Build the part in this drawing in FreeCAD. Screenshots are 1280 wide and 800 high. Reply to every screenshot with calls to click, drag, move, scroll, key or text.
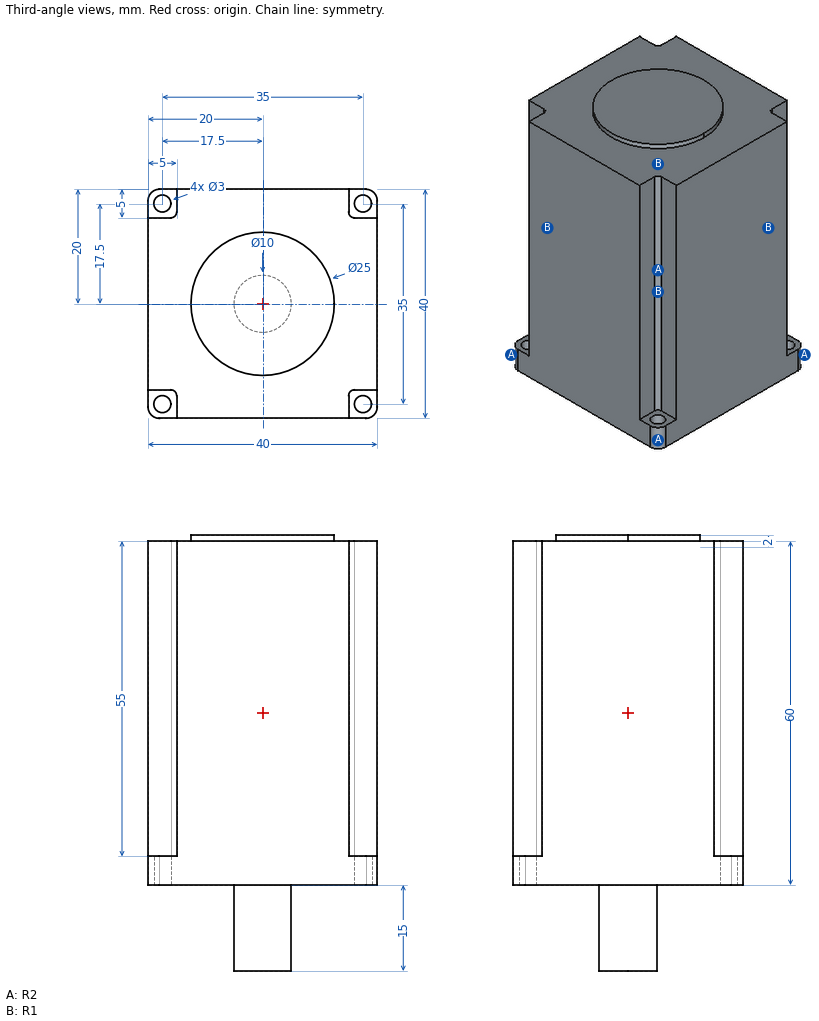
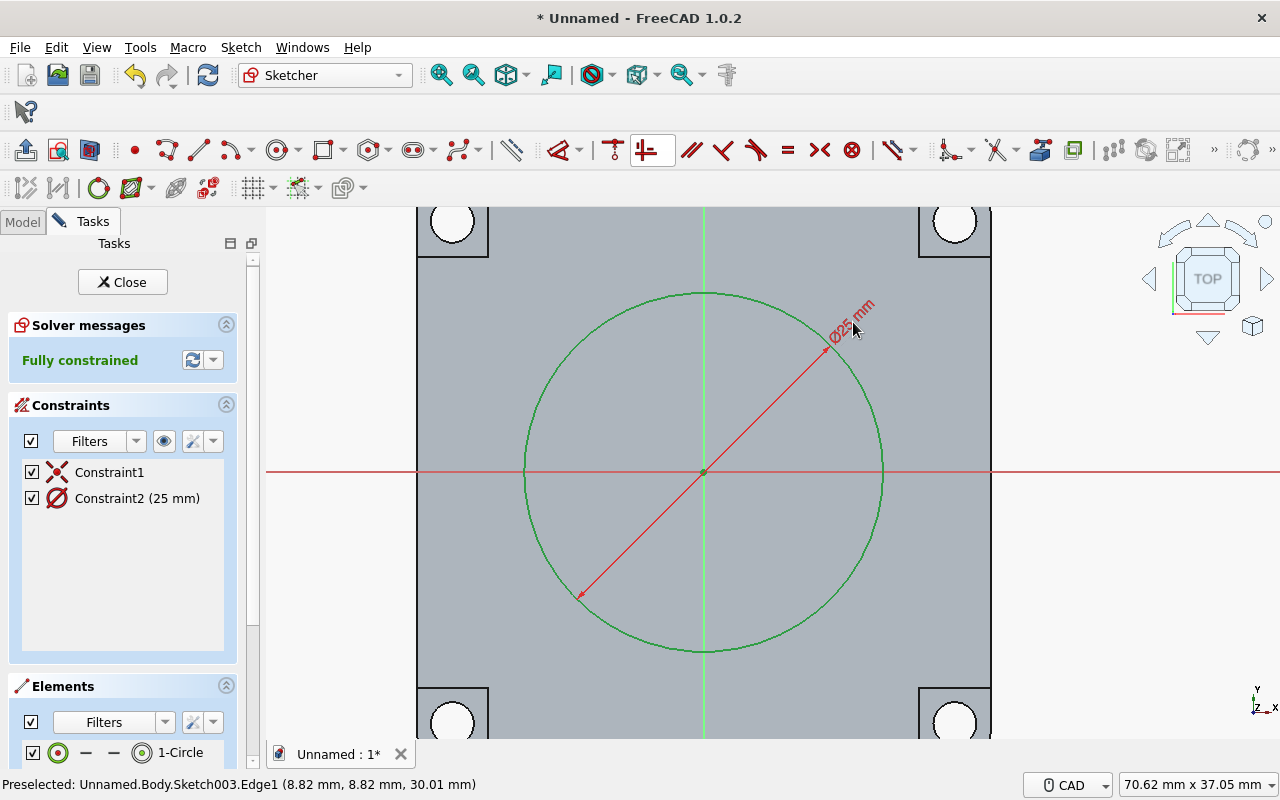
click(123, 282)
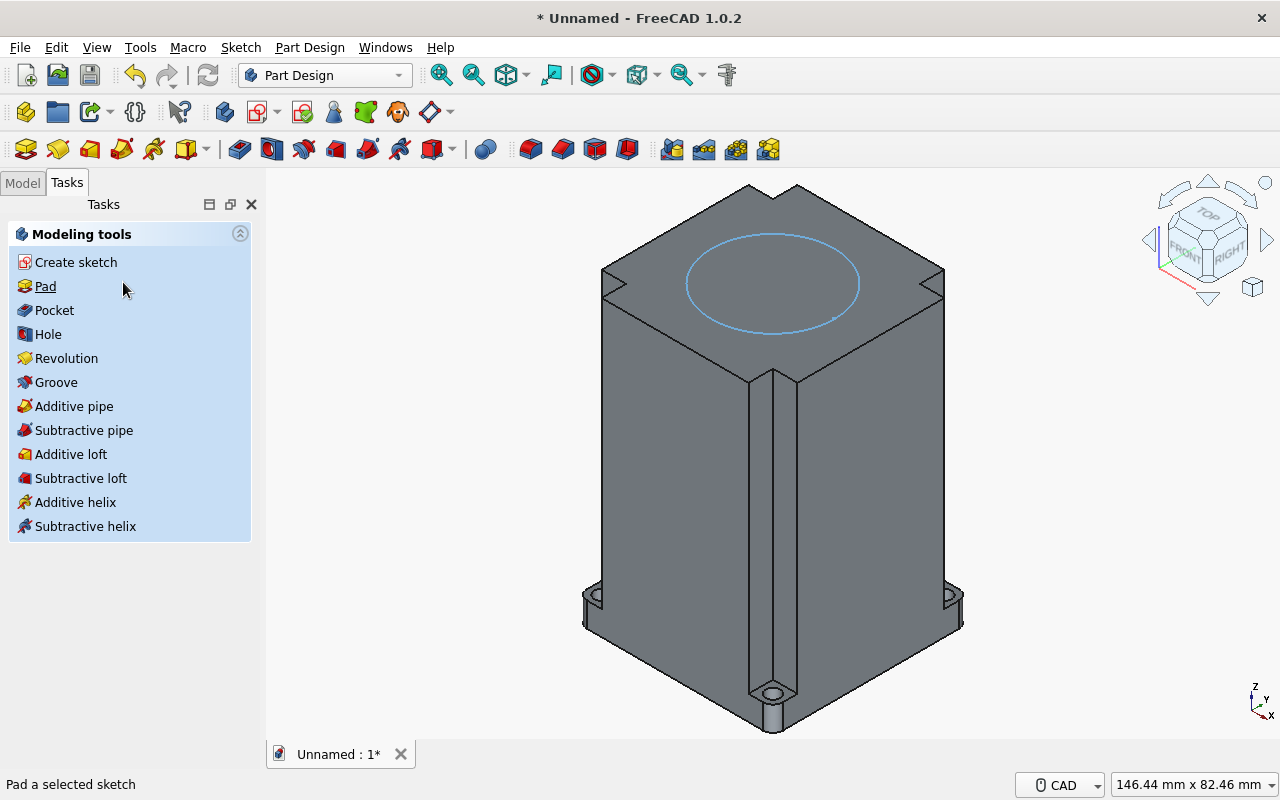
click(26, 150)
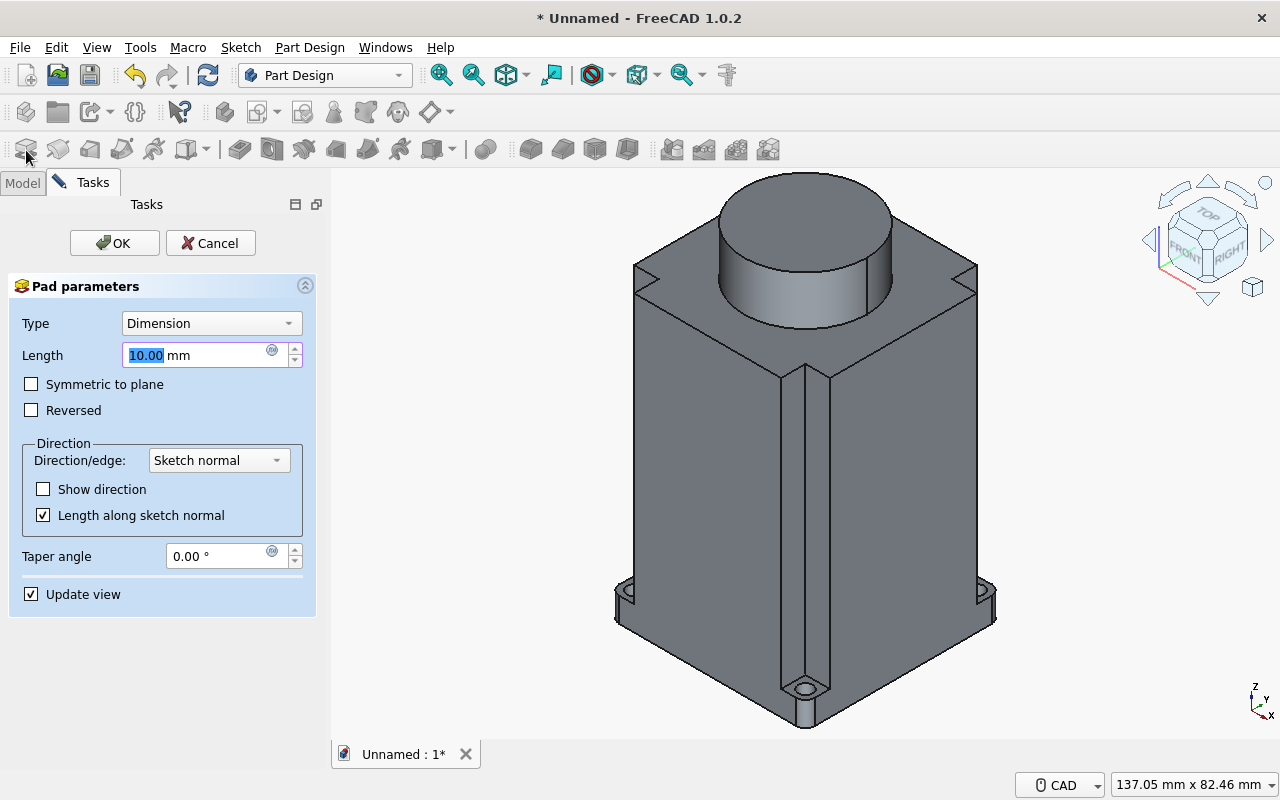
text(2)
key(Tab)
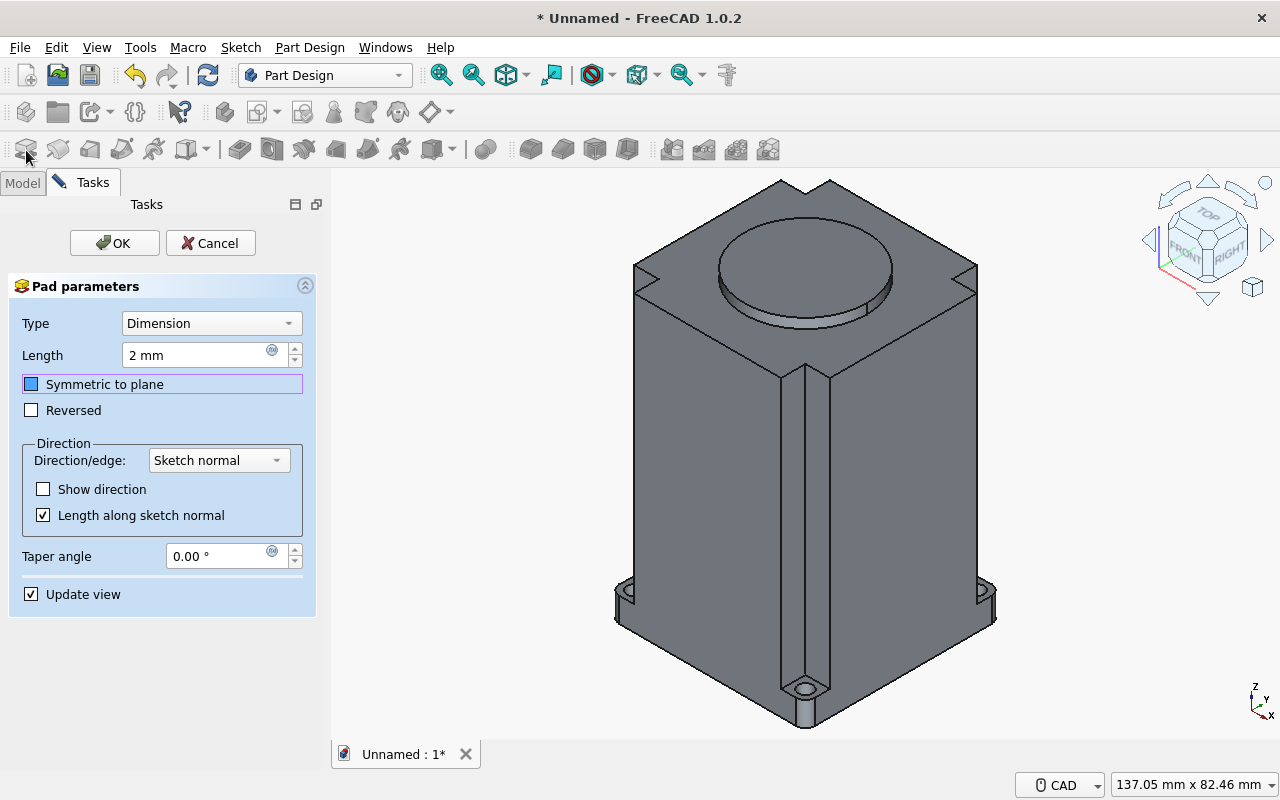
click(30, 384)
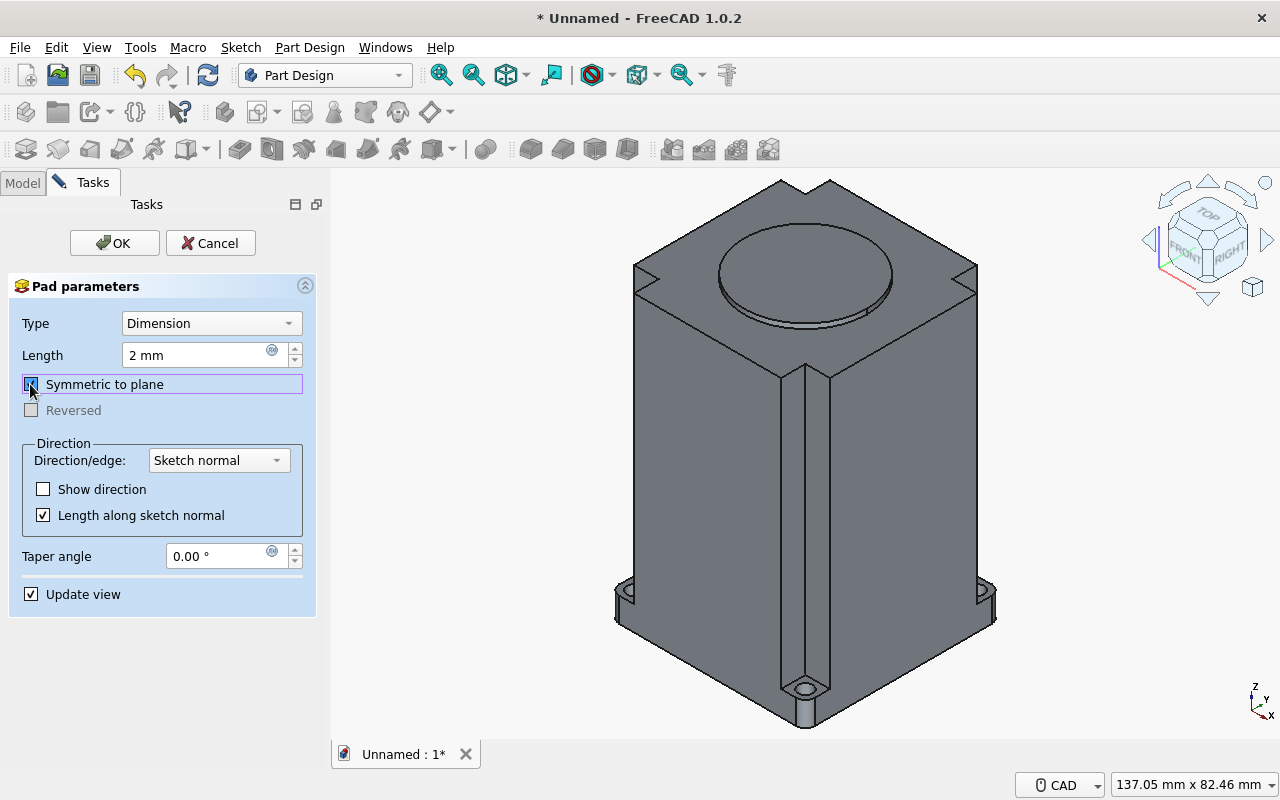
click(115, 243)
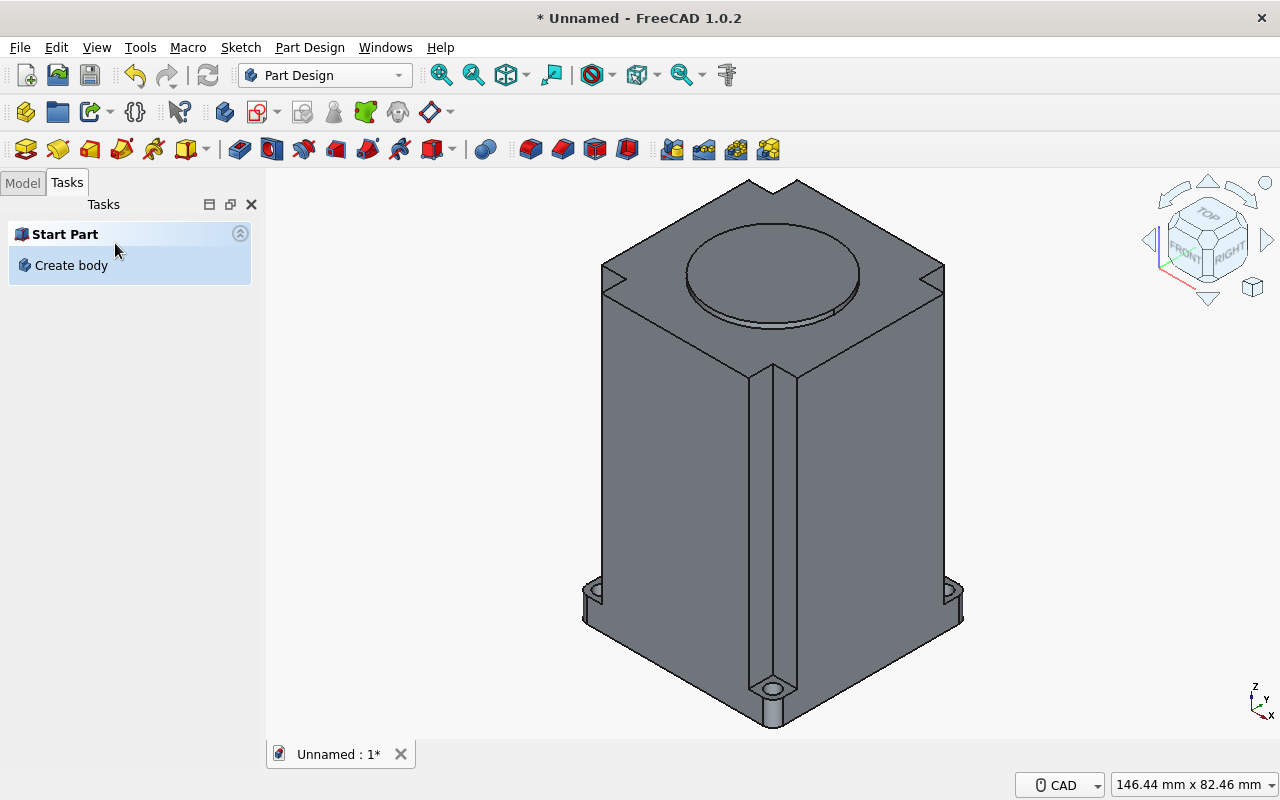
click(442, 76)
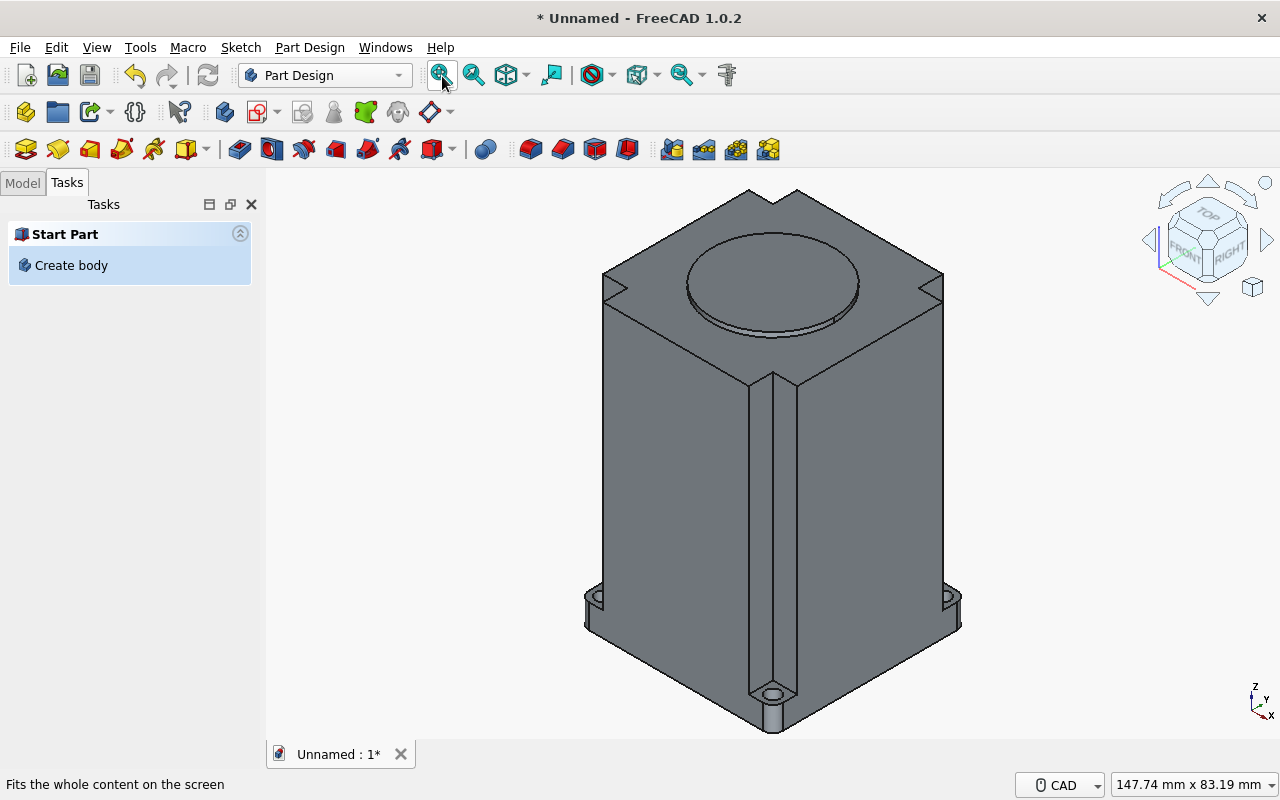
key(2)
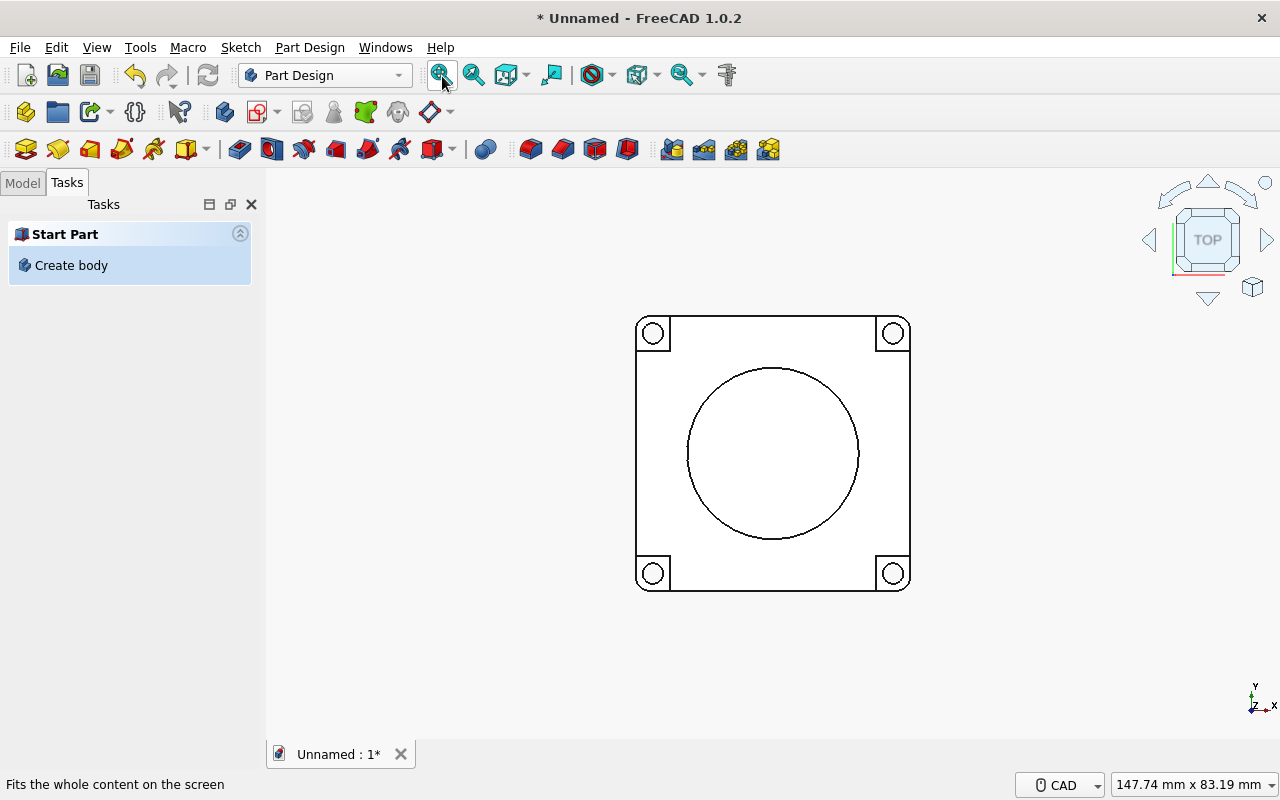
key(0)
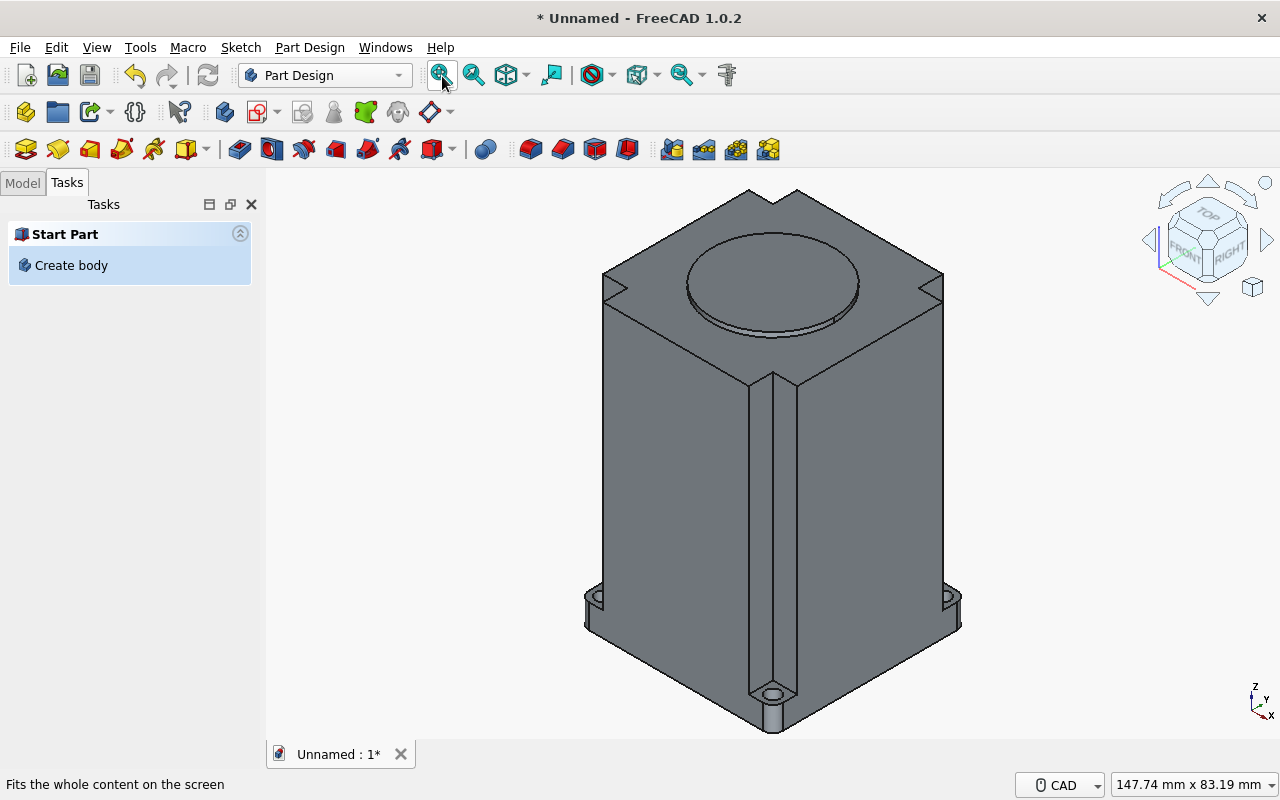
key(1)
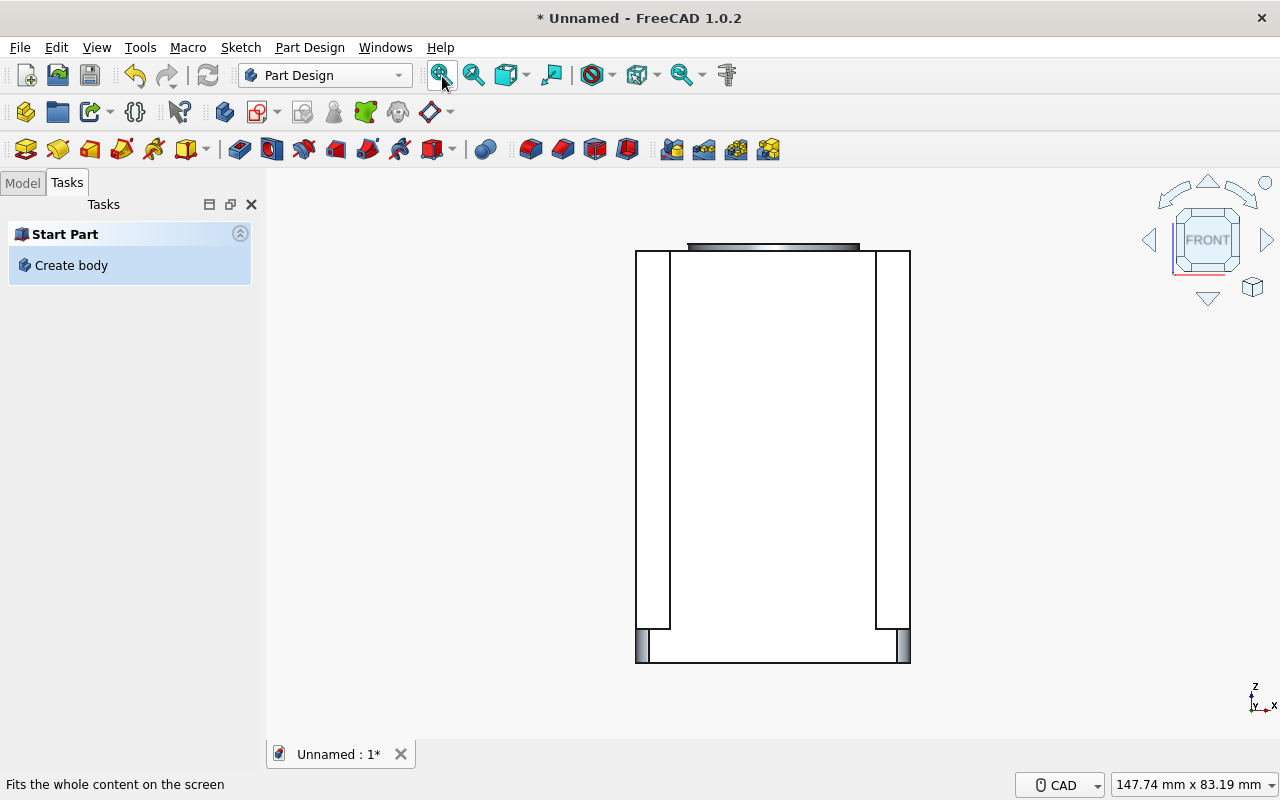
key(3)